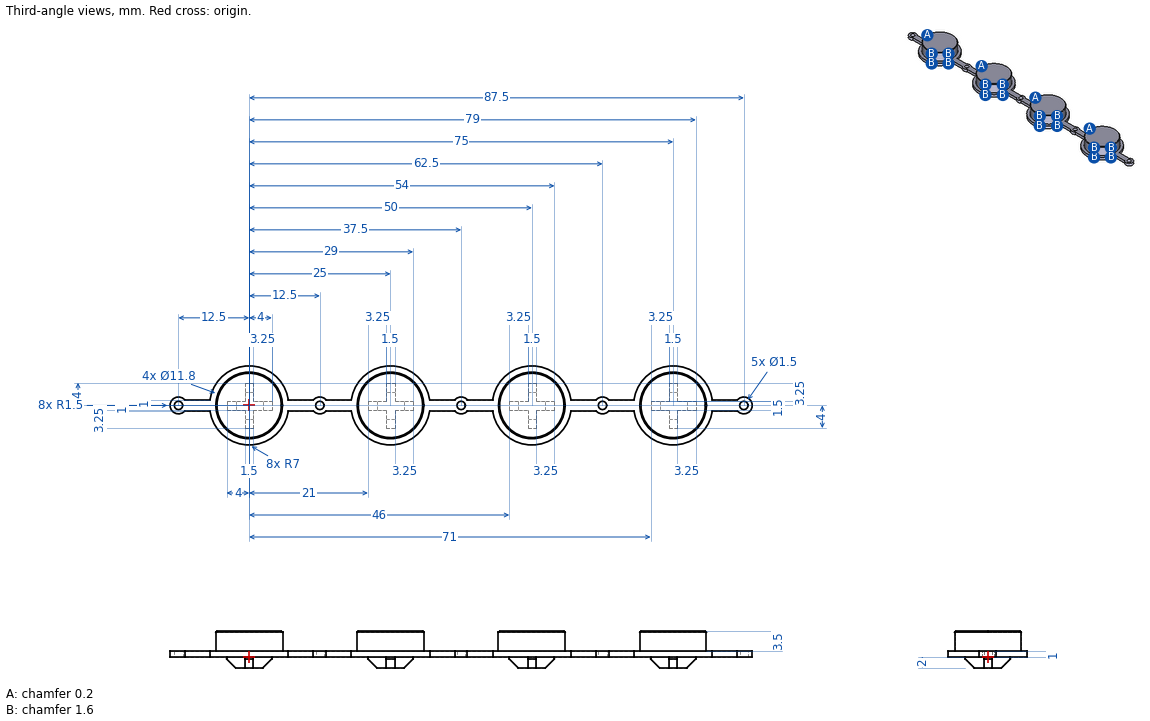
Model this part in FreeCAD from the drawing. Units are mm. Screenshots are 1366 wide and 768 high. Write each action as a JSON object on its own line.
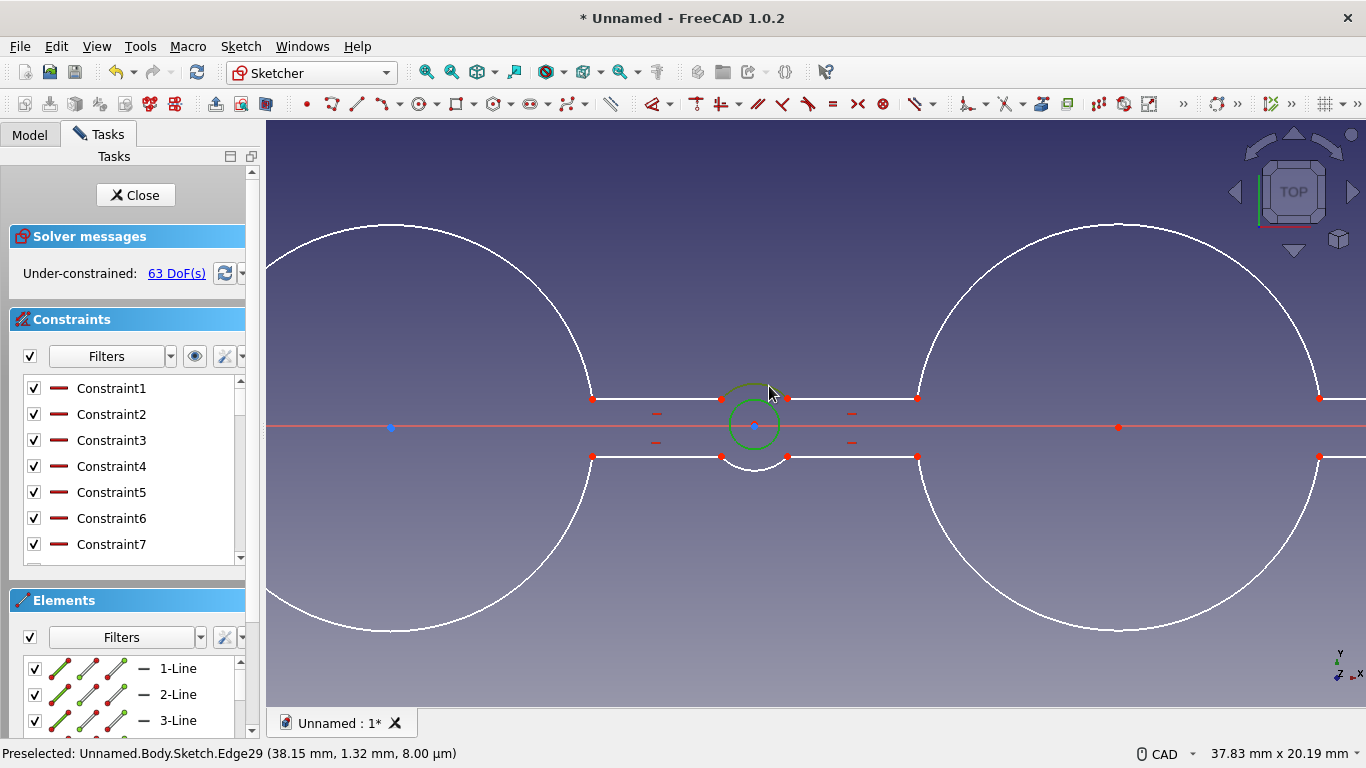
{"action": "left_click", "coordinate": [696, 104]}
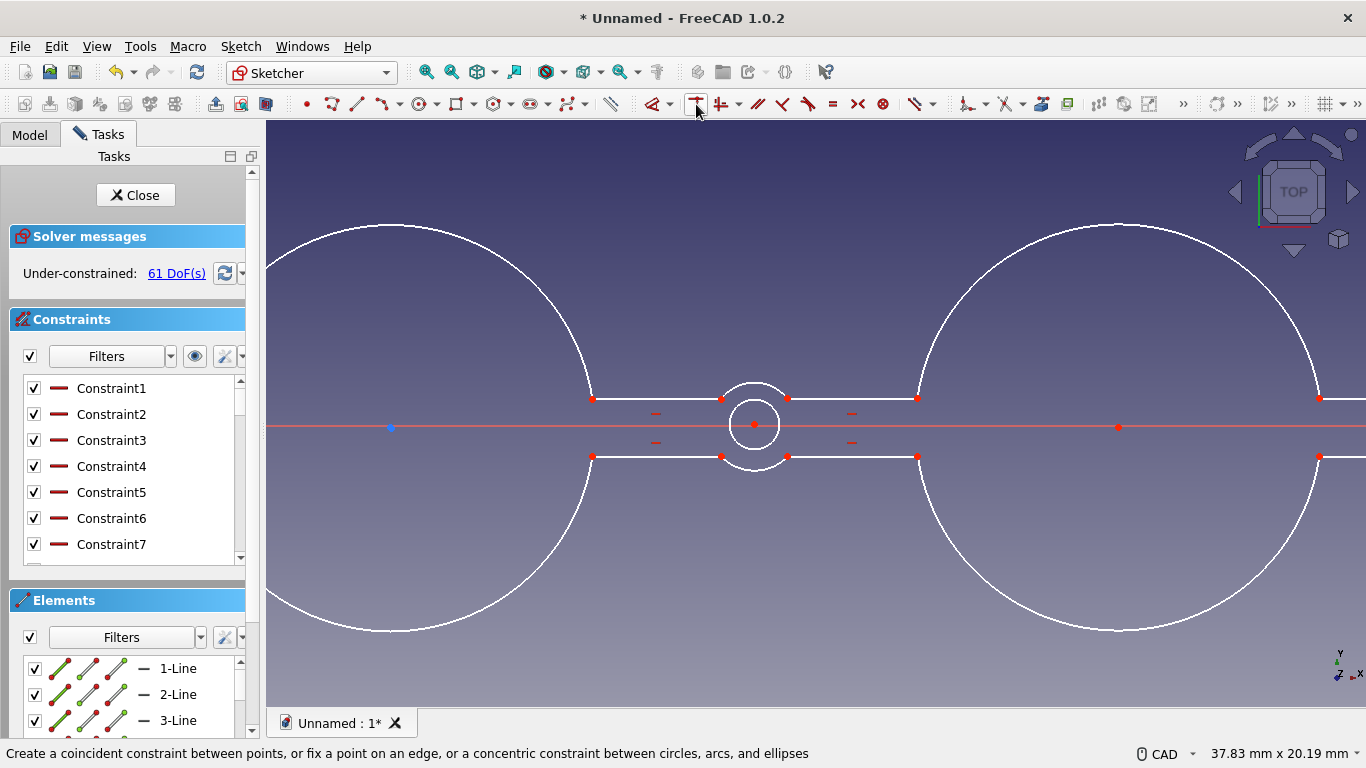
{"action": "scroll", "coordinate": [746, 410], "scroll_direction": "down", "scroll_amount": 8}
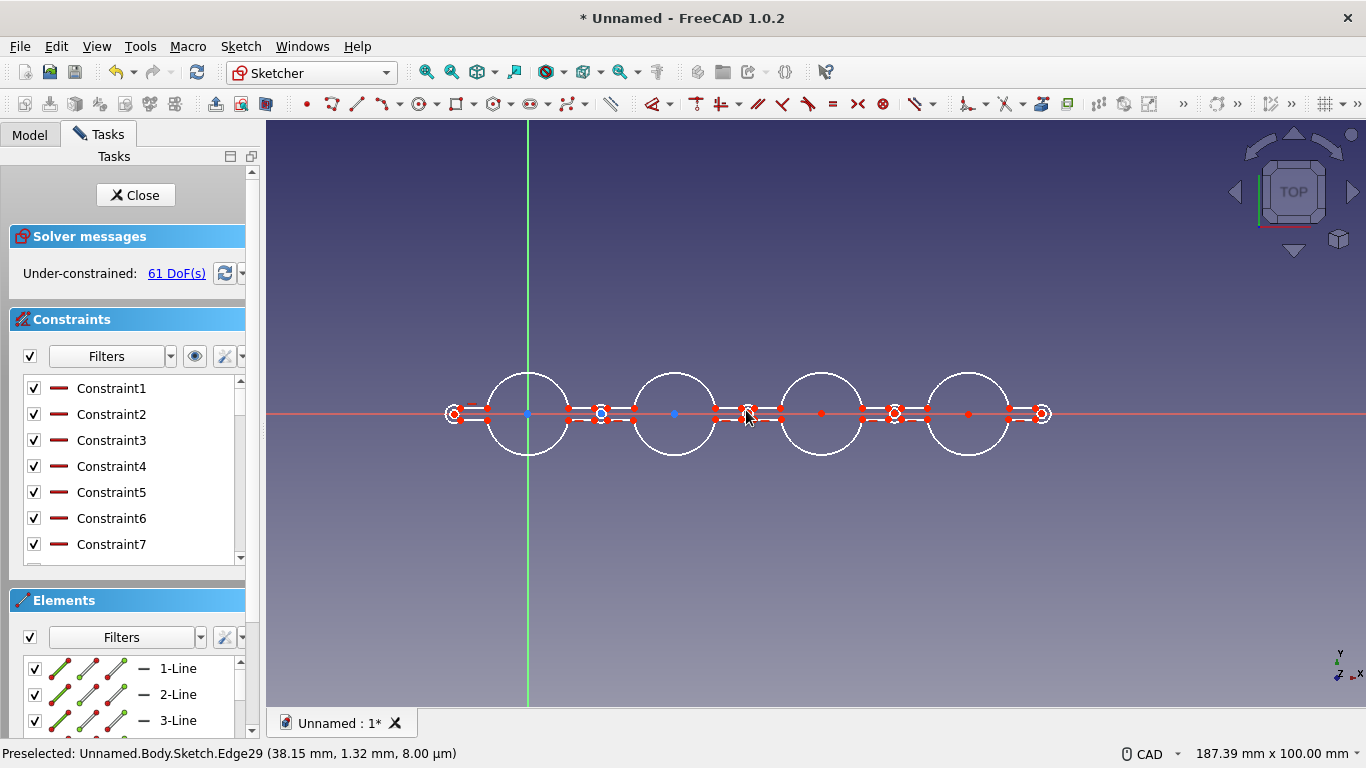
{"action": "left_click", "coordinate": [697, 449]}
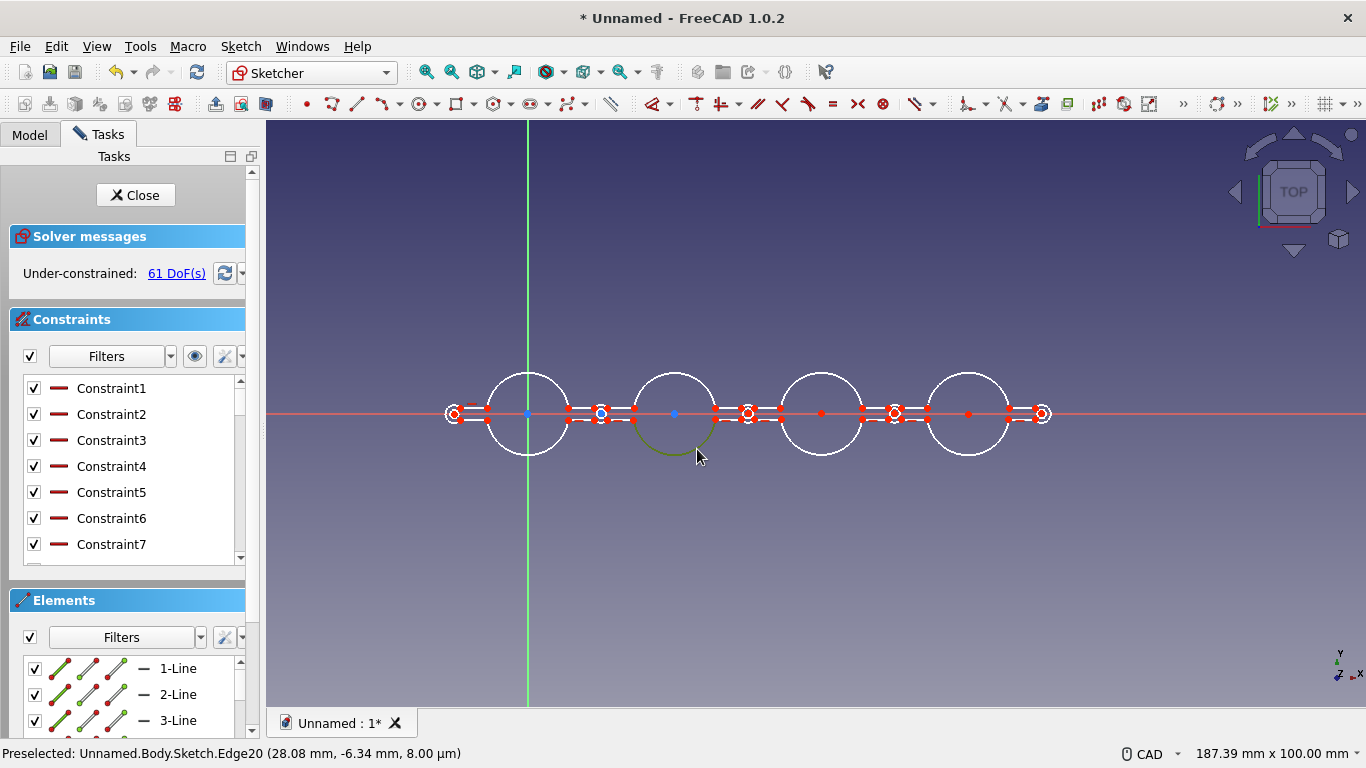
{"action": "left_click", "coordinate": [697, 380]}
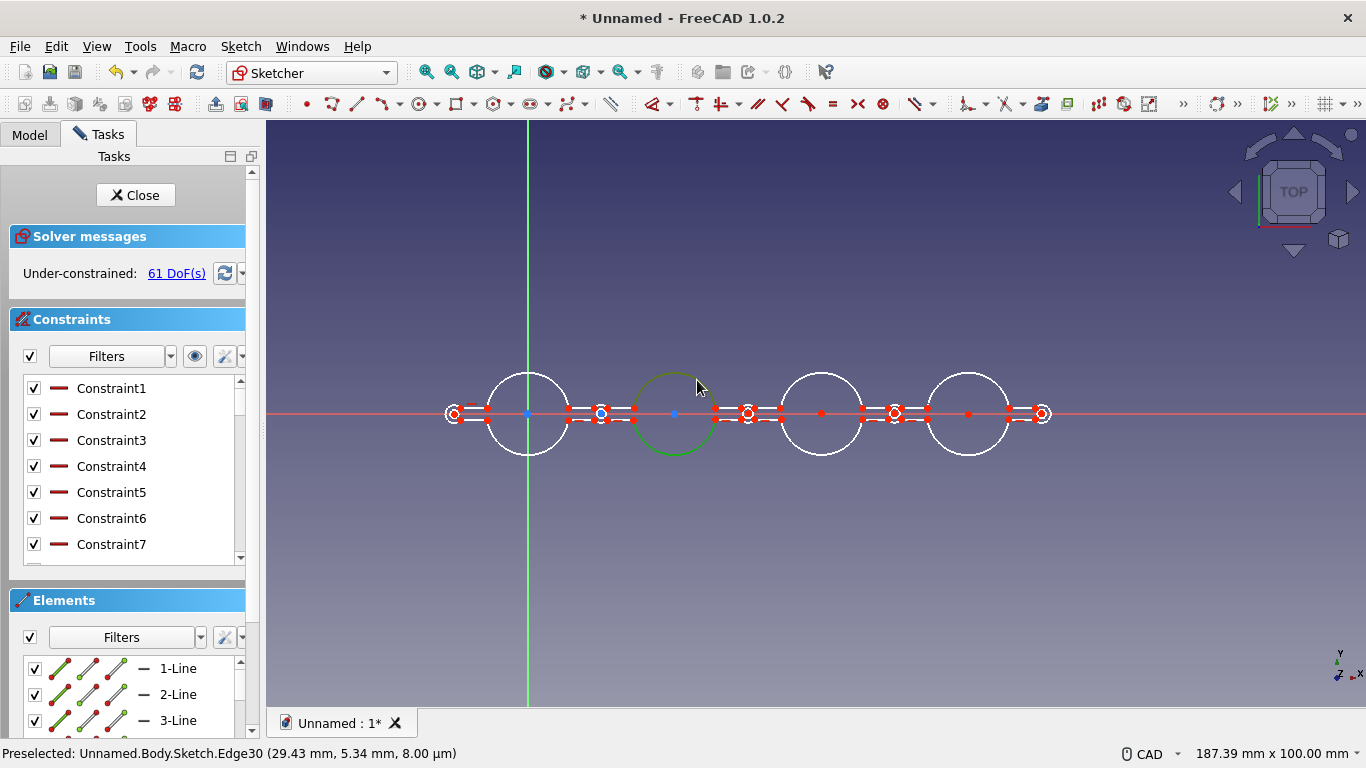
{"action": "key", "text": "c"}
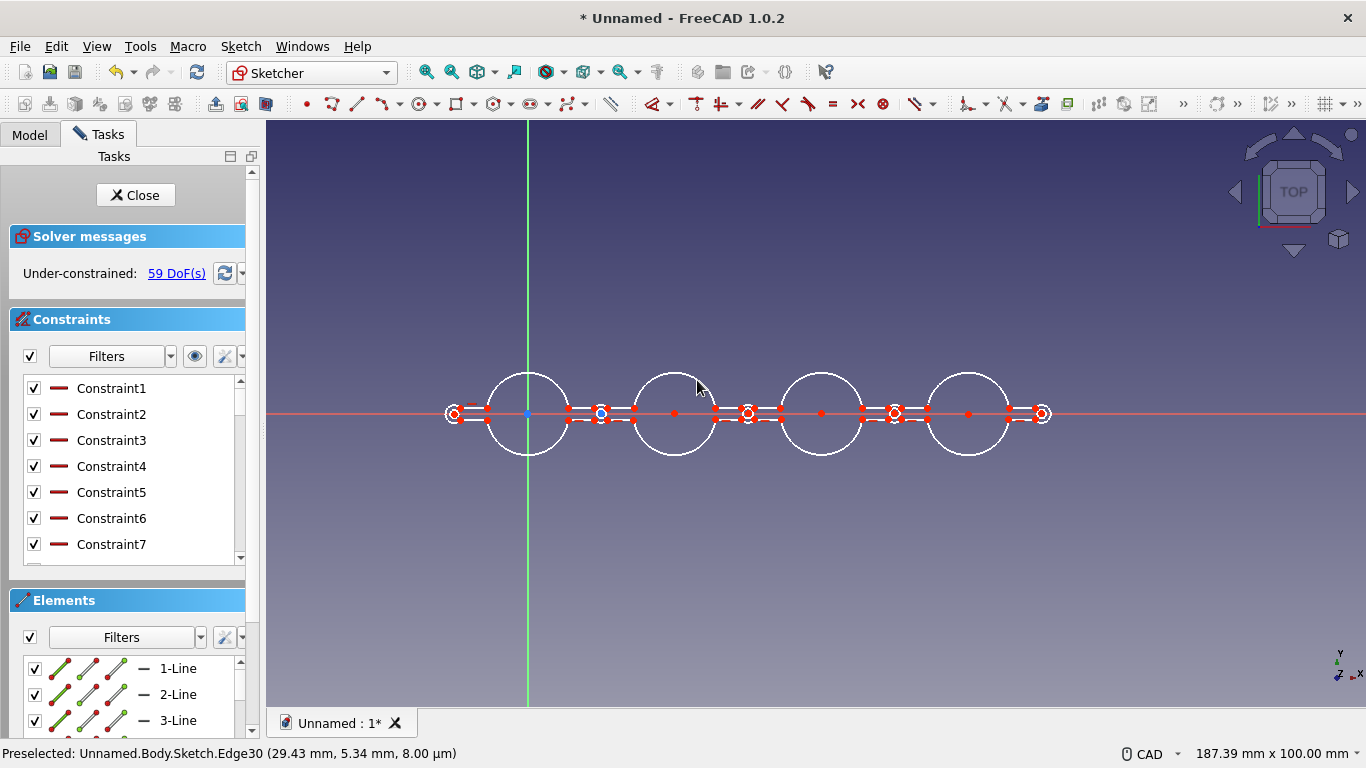
{"action": "scroll", "coordinate": [597, 414], "scroll_direction": "up", "scroll_amount": 6}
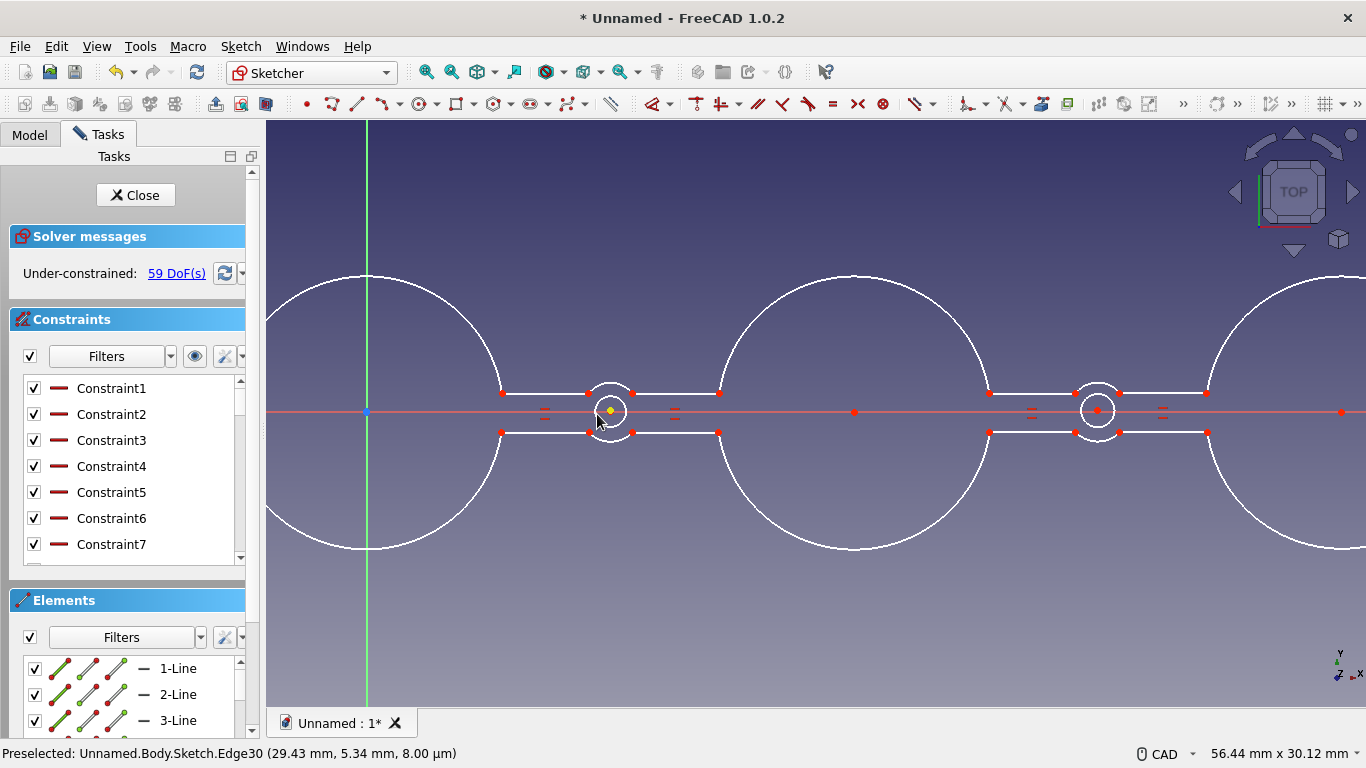
{"action": "left_click", "coordinate": [595, 411]}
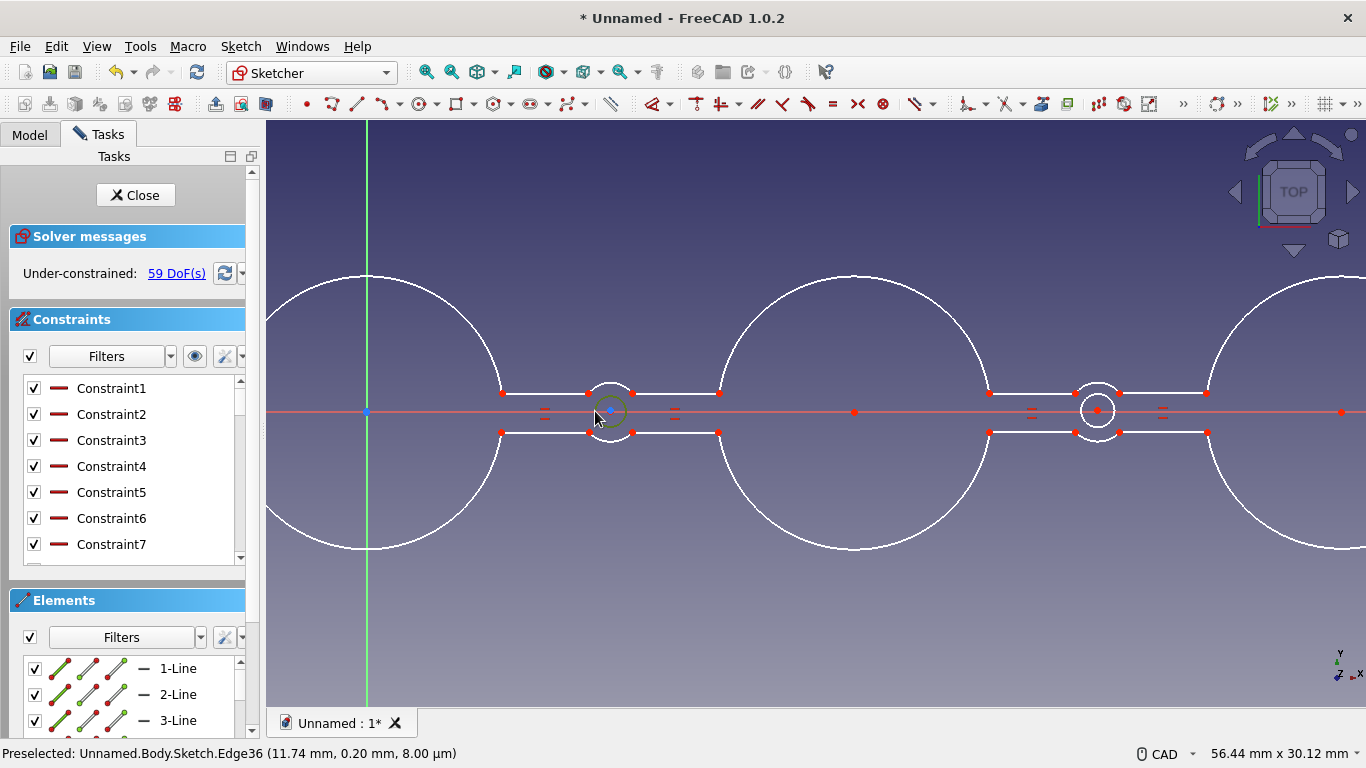
{"action": "left_click", "coordinate": [621, 385]}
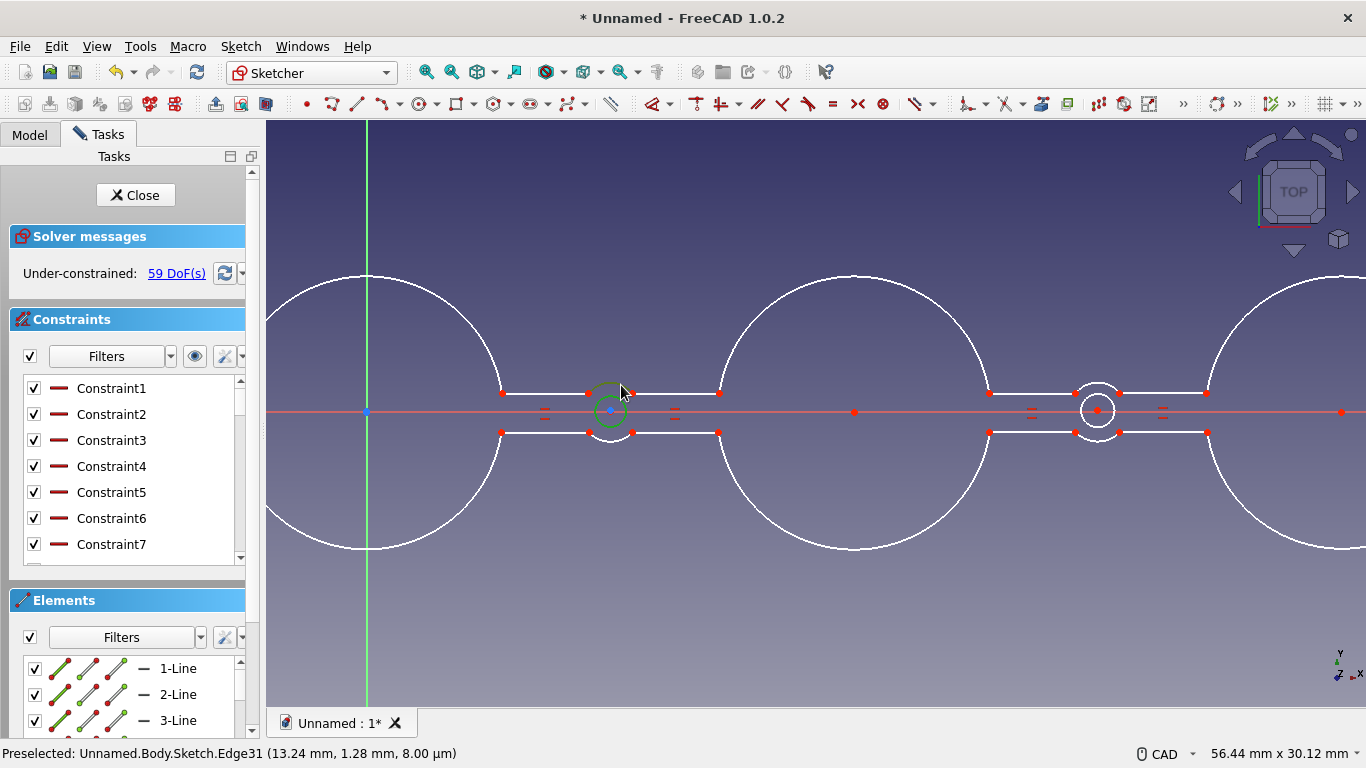
{"action": "key", "text": "c"}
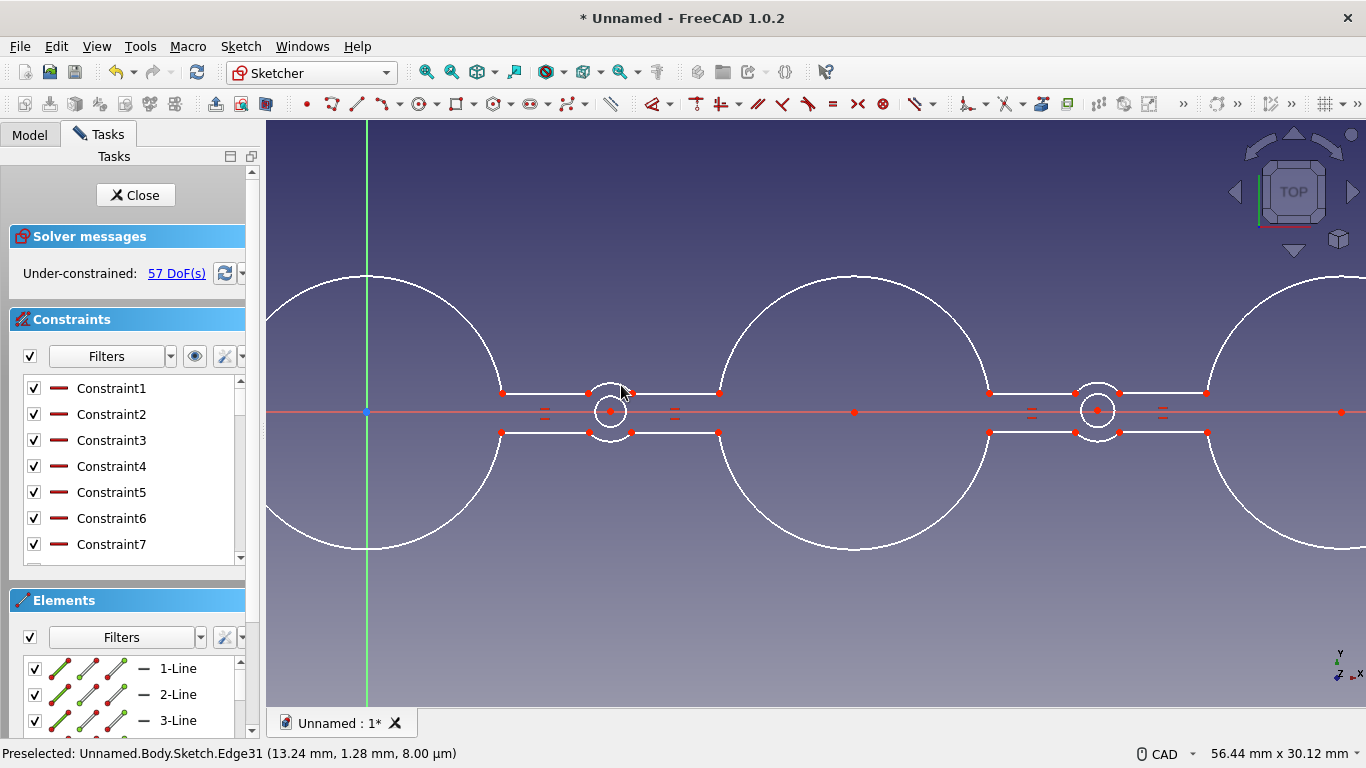
{"action": "scroll", "coordinate": [597, 414], "scroll_direction": "down", "scroll_amount": 6}